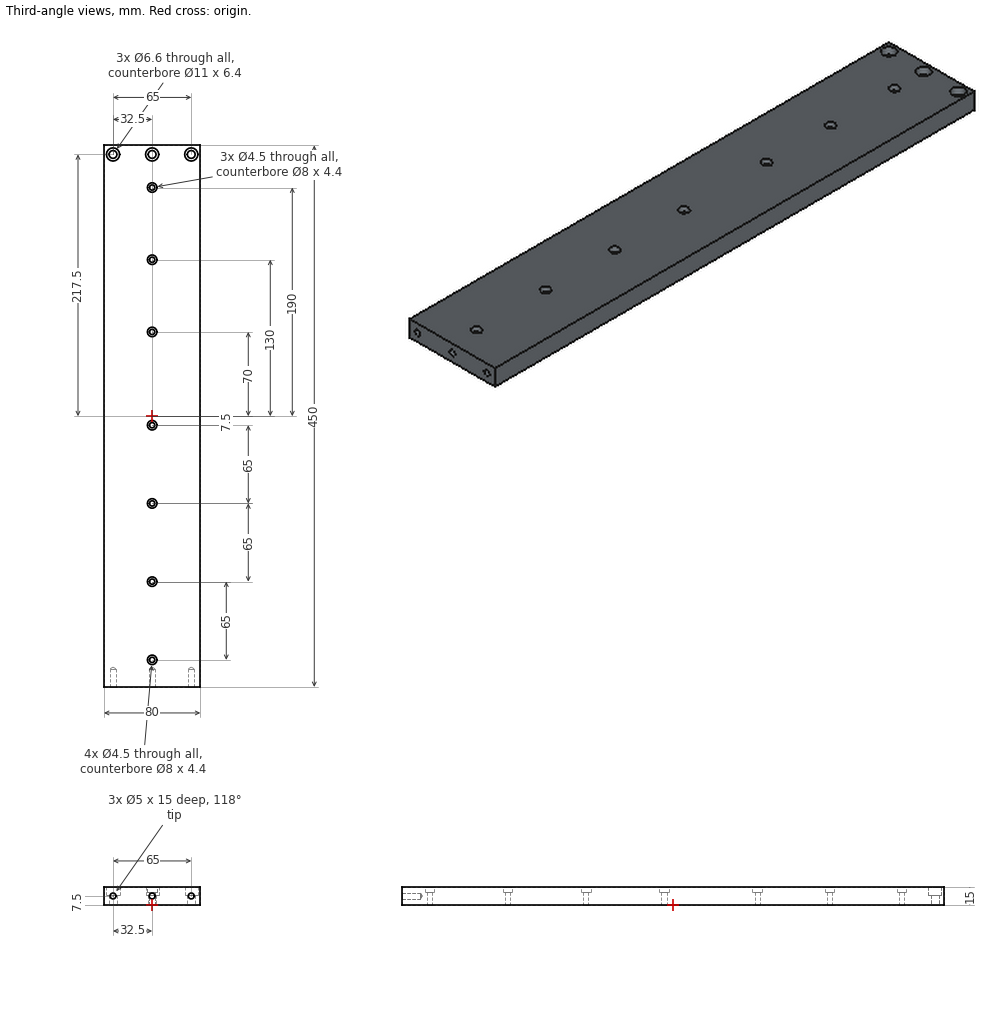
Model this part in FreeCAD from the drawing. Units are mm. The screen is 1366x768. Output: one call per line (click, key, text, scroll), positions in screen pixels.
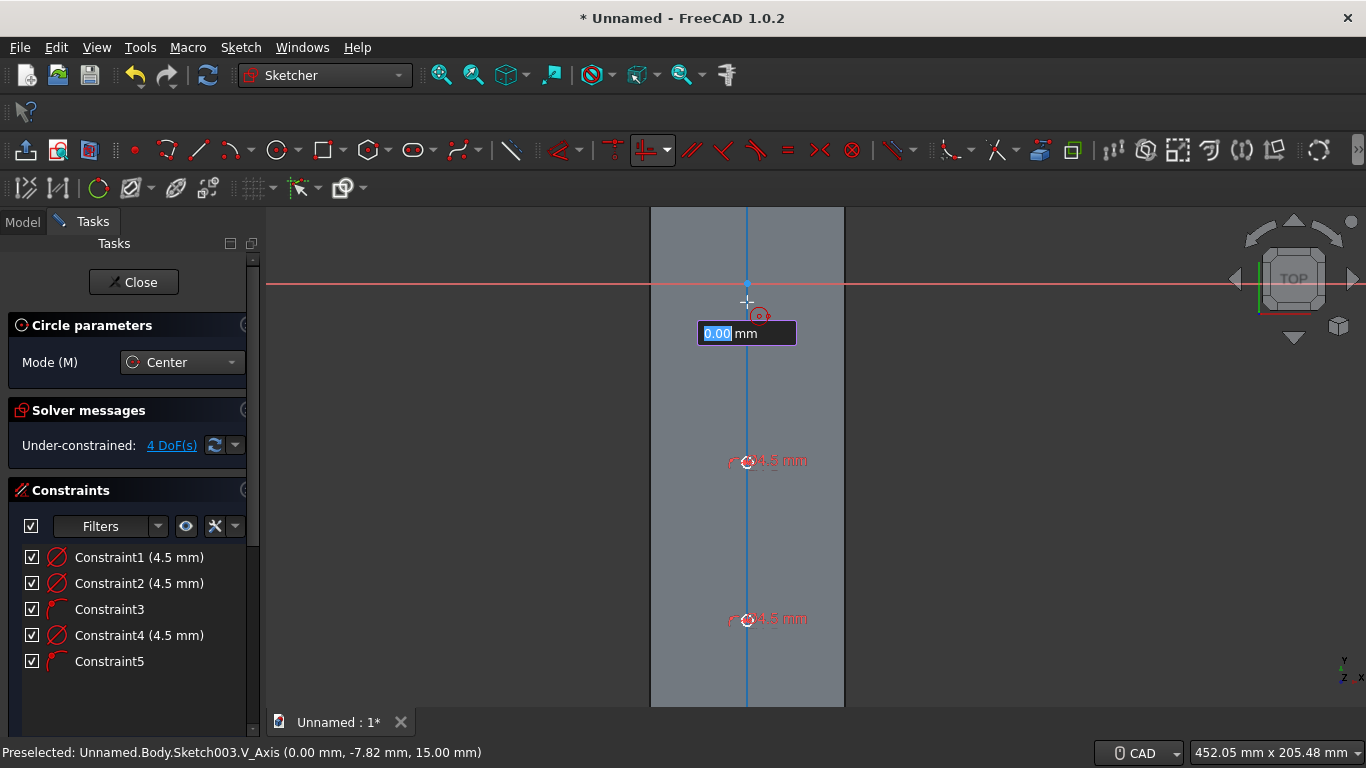
scroll(752, 300, up, 6)
move(752, 301)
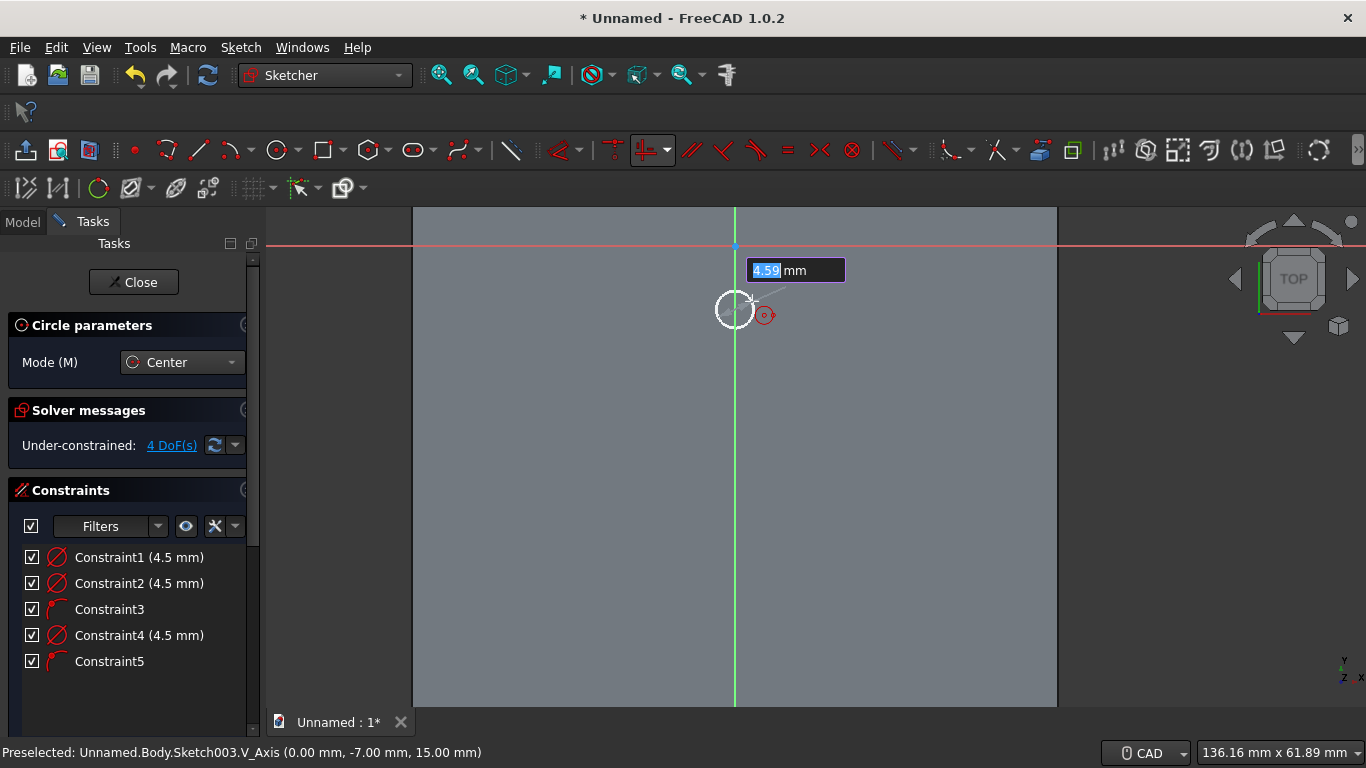
text(4.5)
key(Return)
key(Escape)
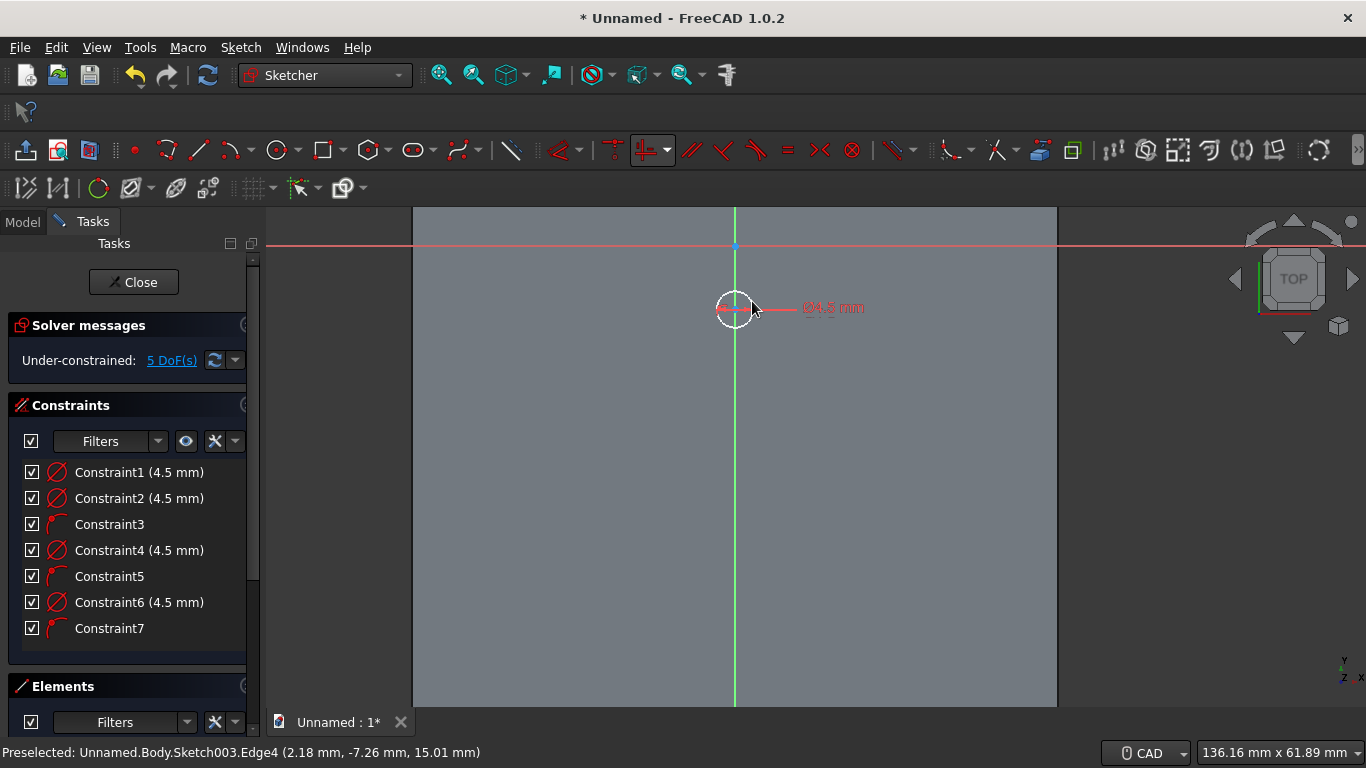
scroll(751, 301, down, 8)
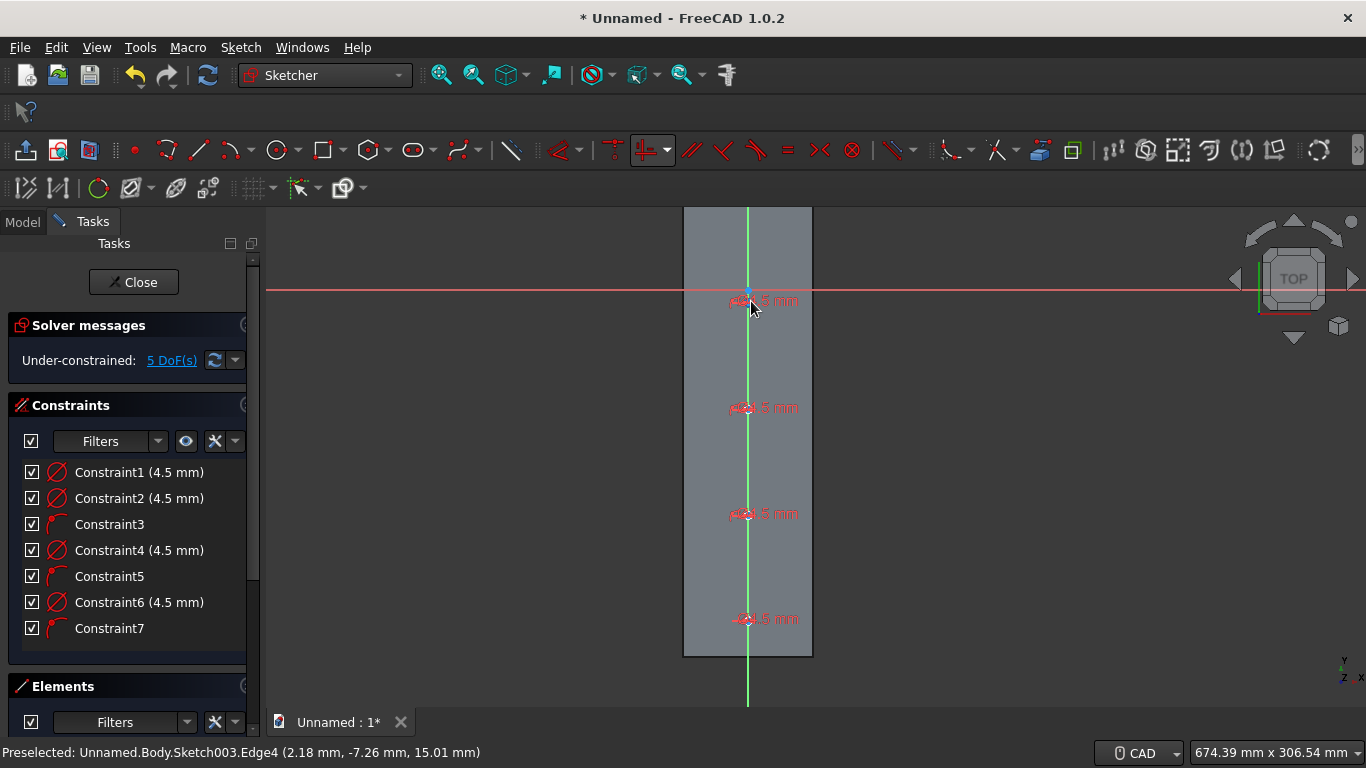
click(749, 621)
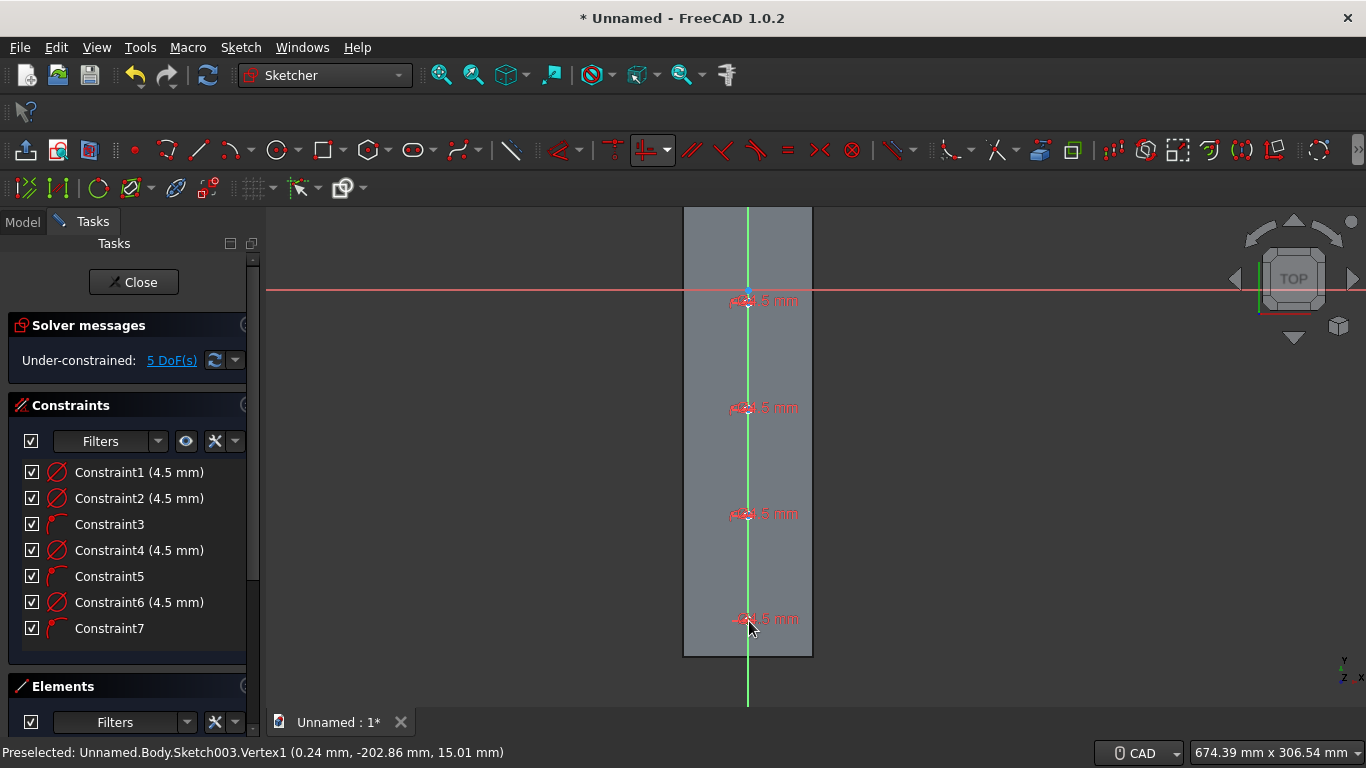
click(748, 584)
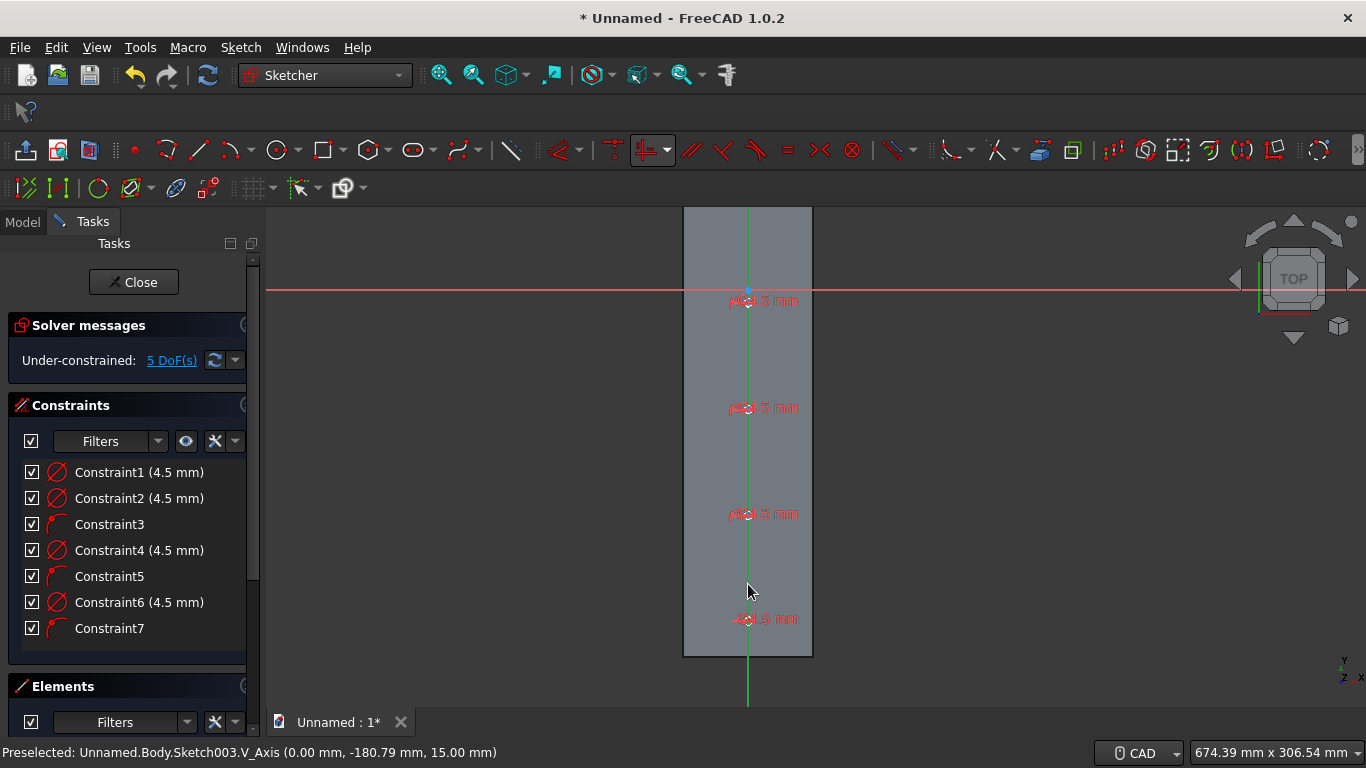
click(614, 150)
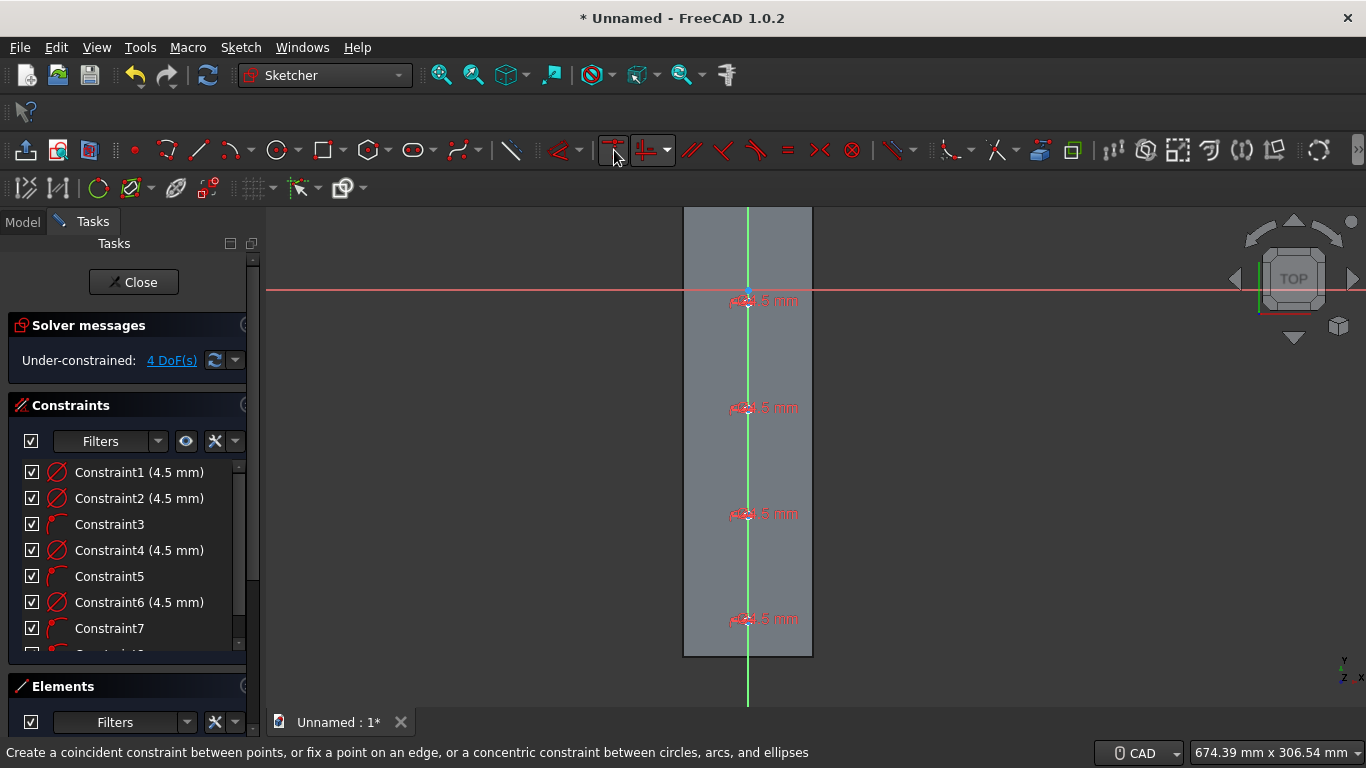
click(558, 150)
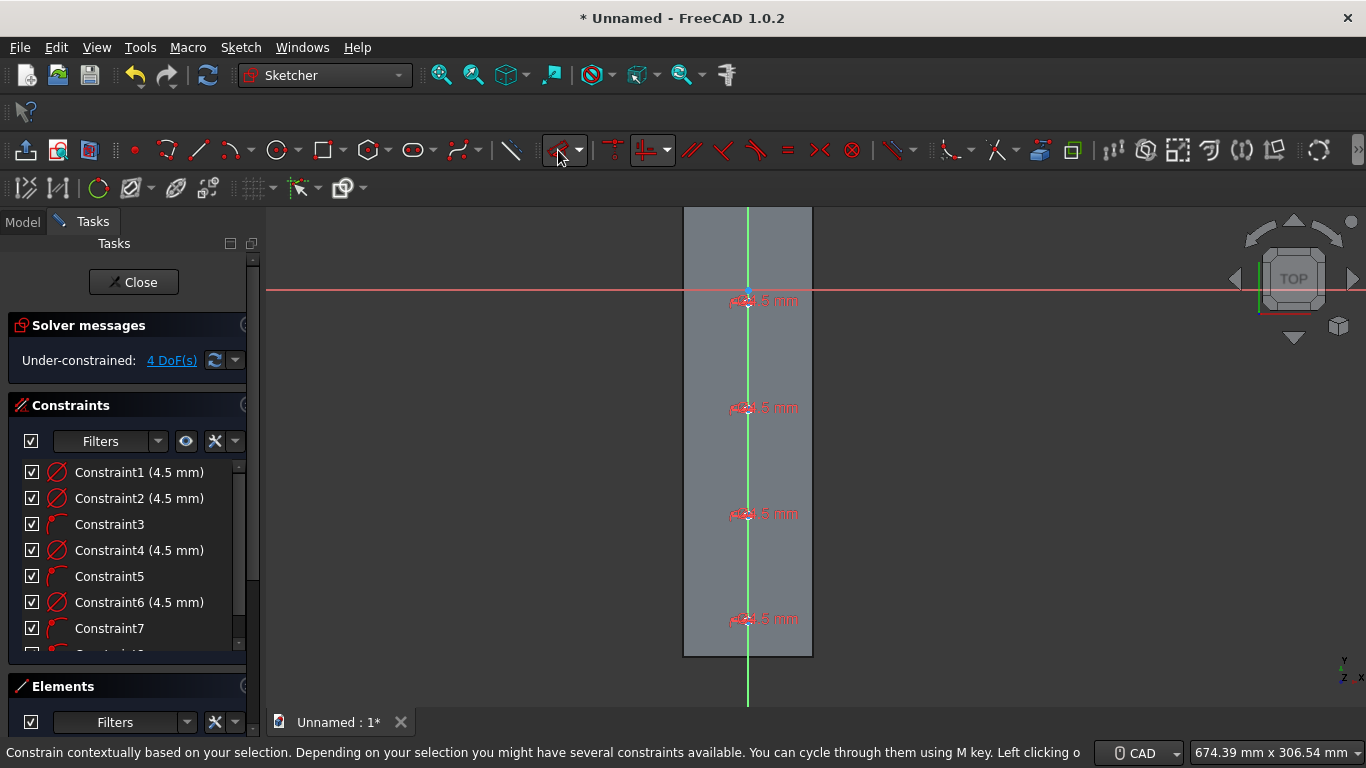
scroll(748, 303, up, 6)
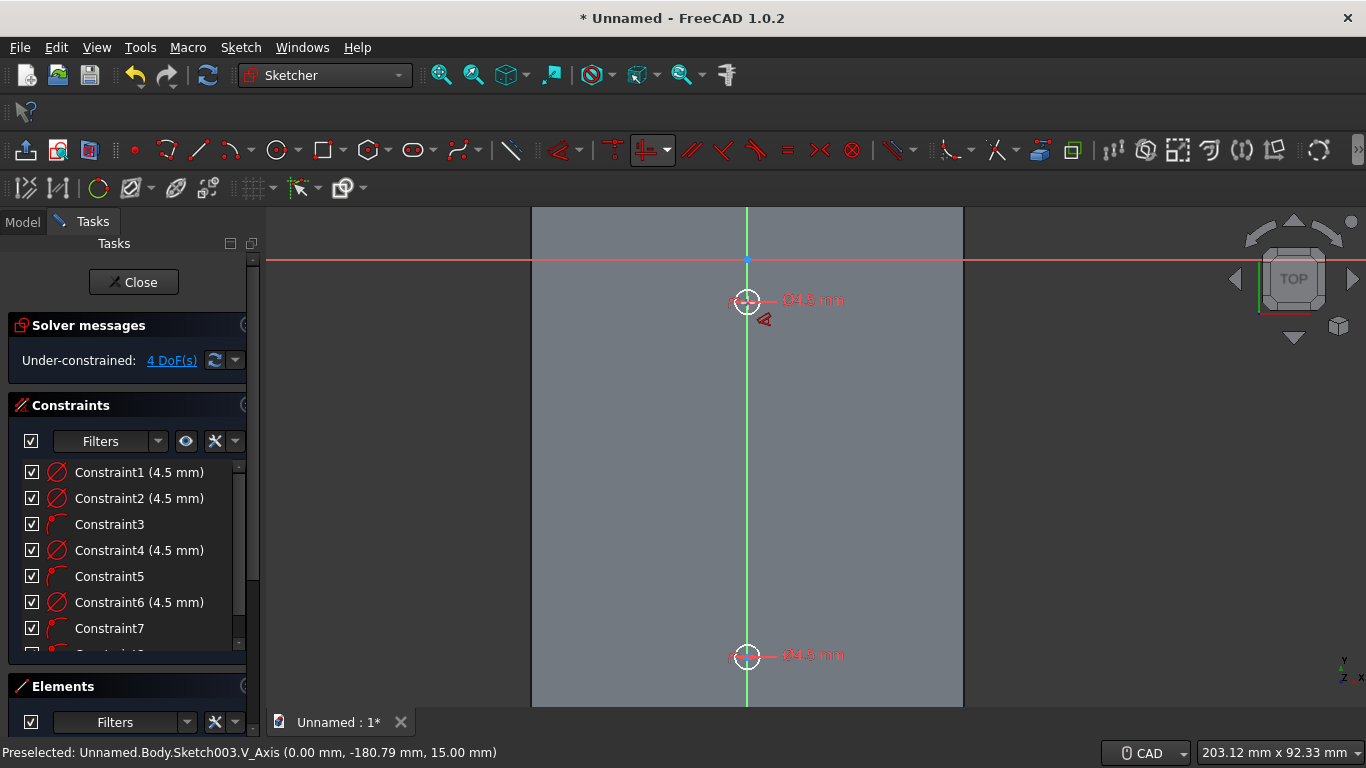
click(747, 302)
click(781, 281)